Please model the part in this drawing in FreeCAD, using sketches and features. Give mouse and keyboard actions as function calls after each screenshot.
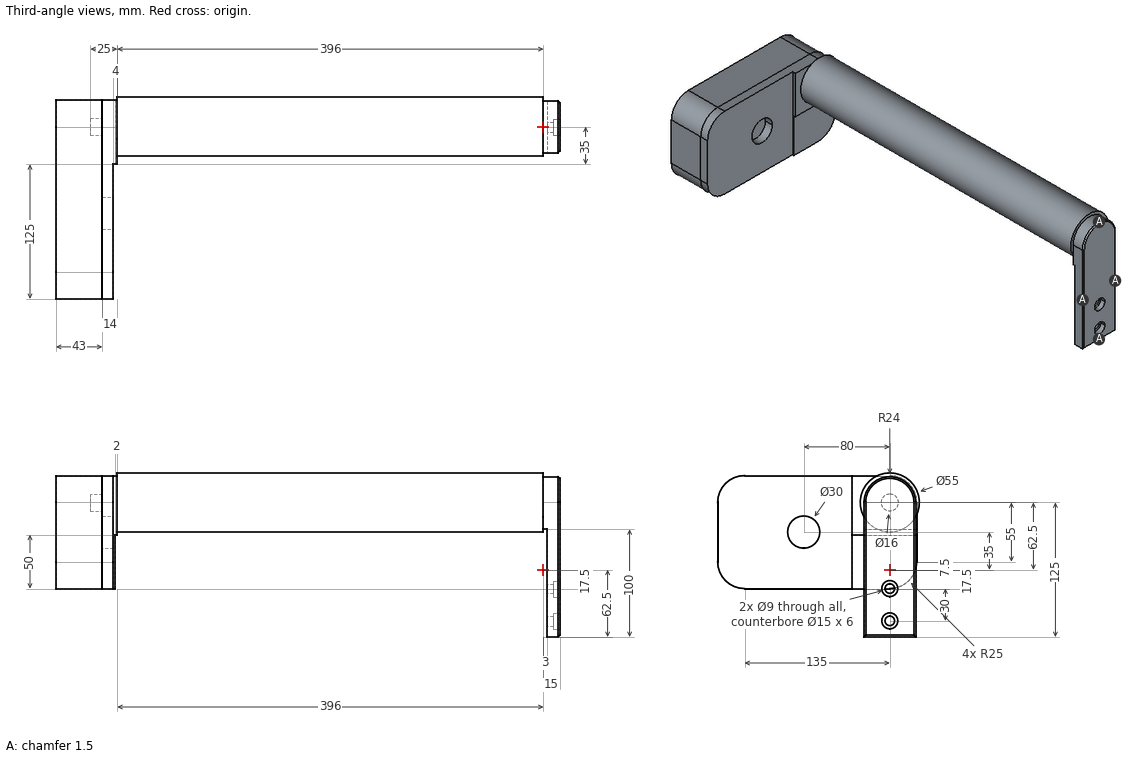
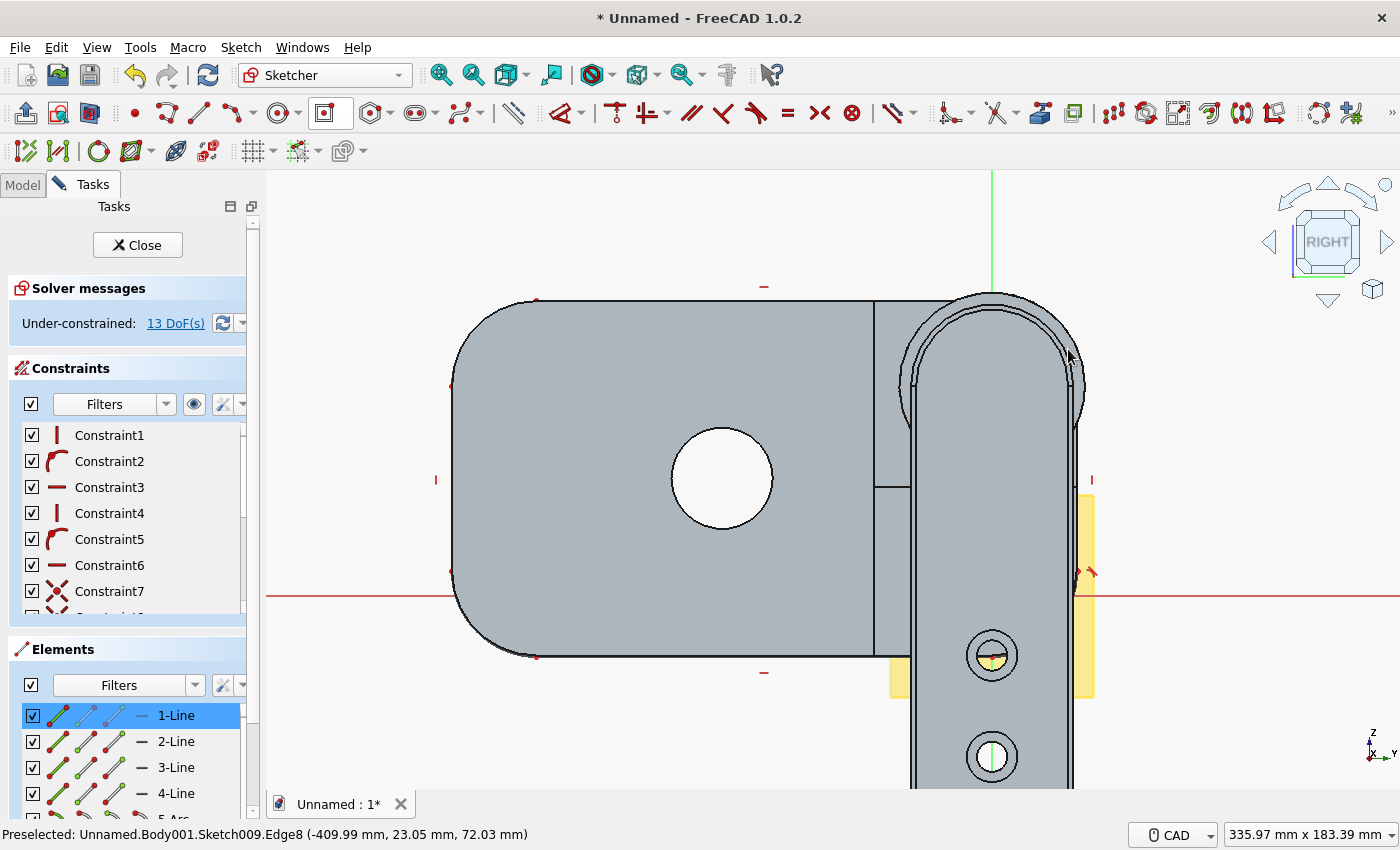
key(t)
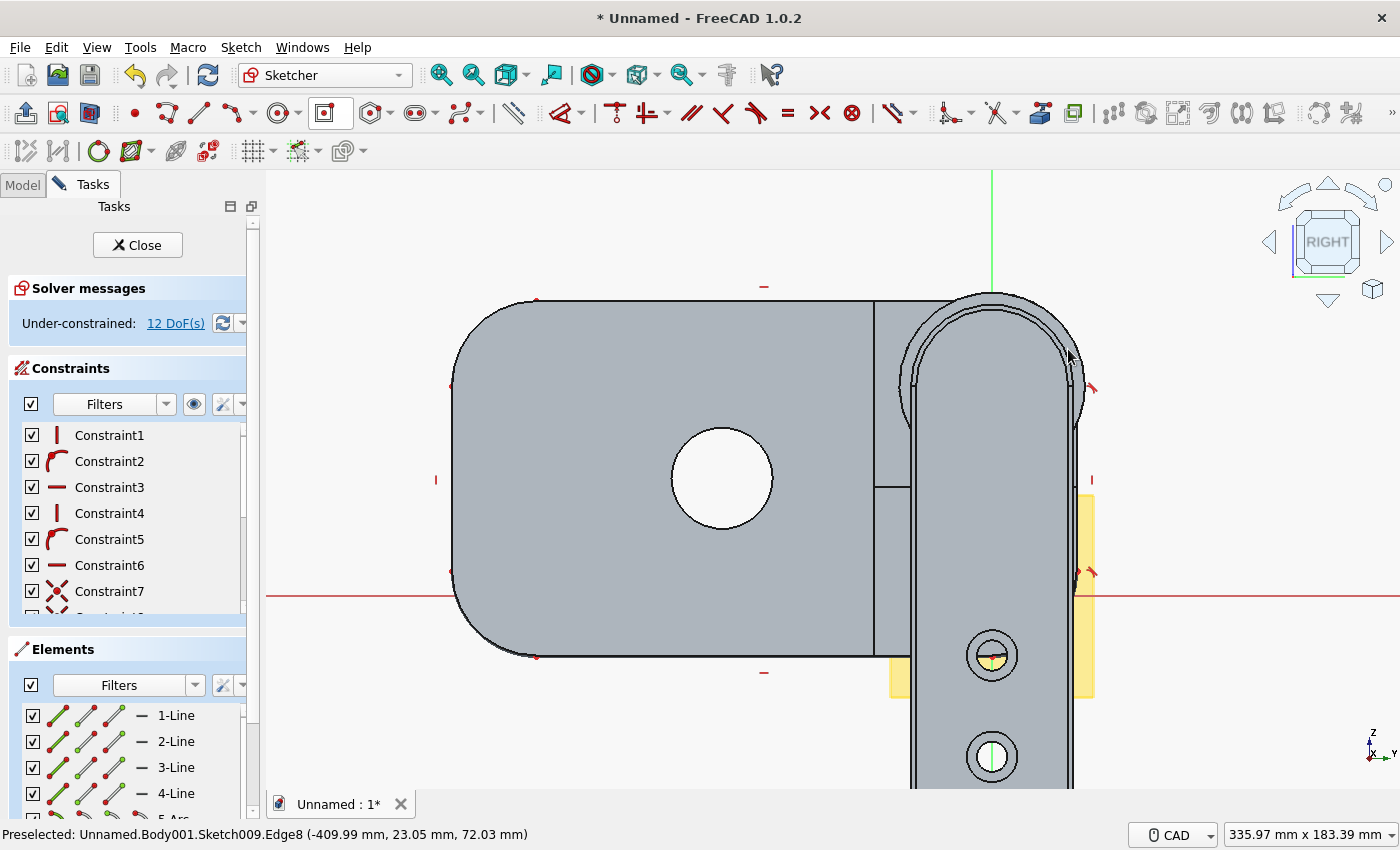
click(855, 657)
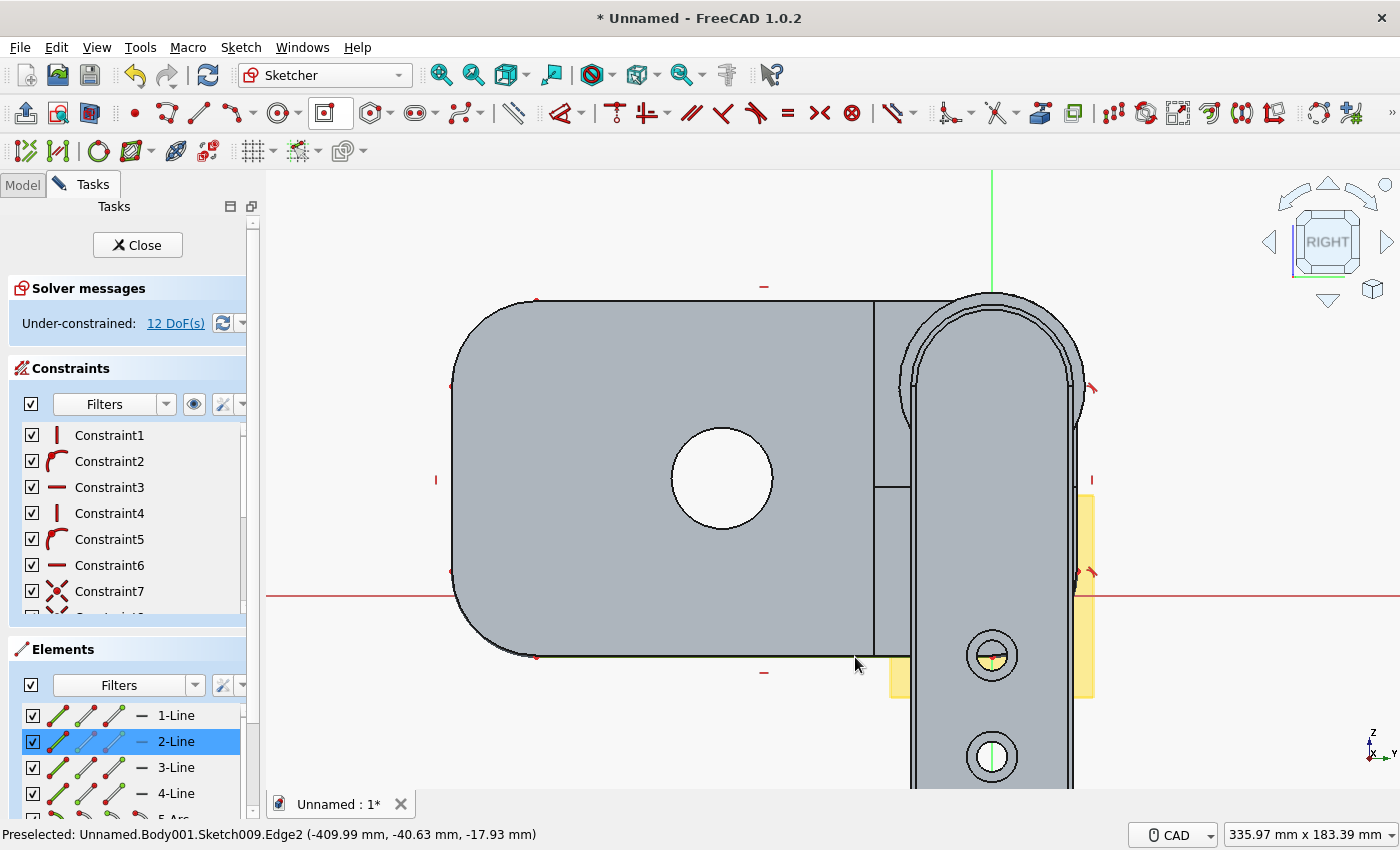
click(1031, 648)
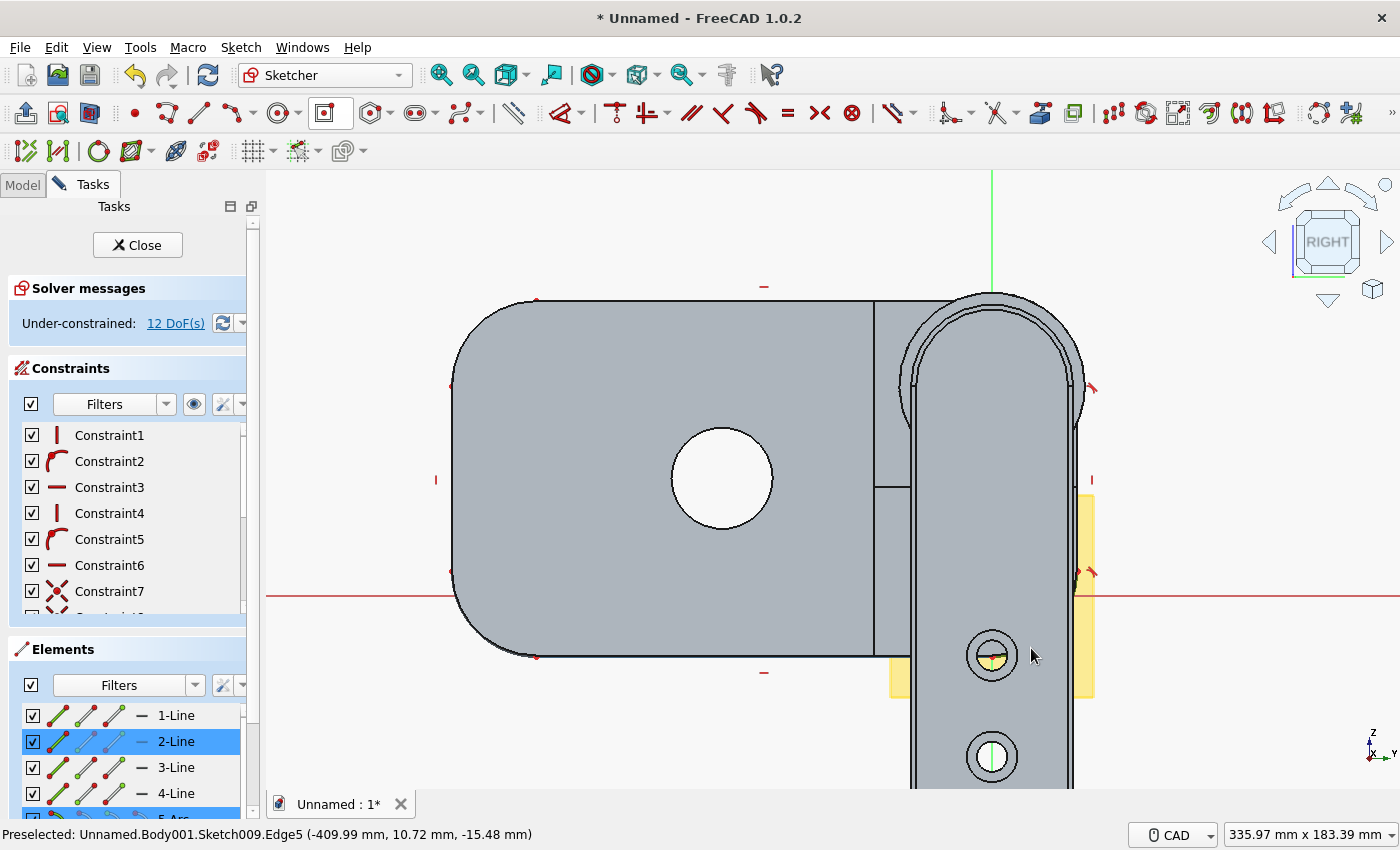
key(t)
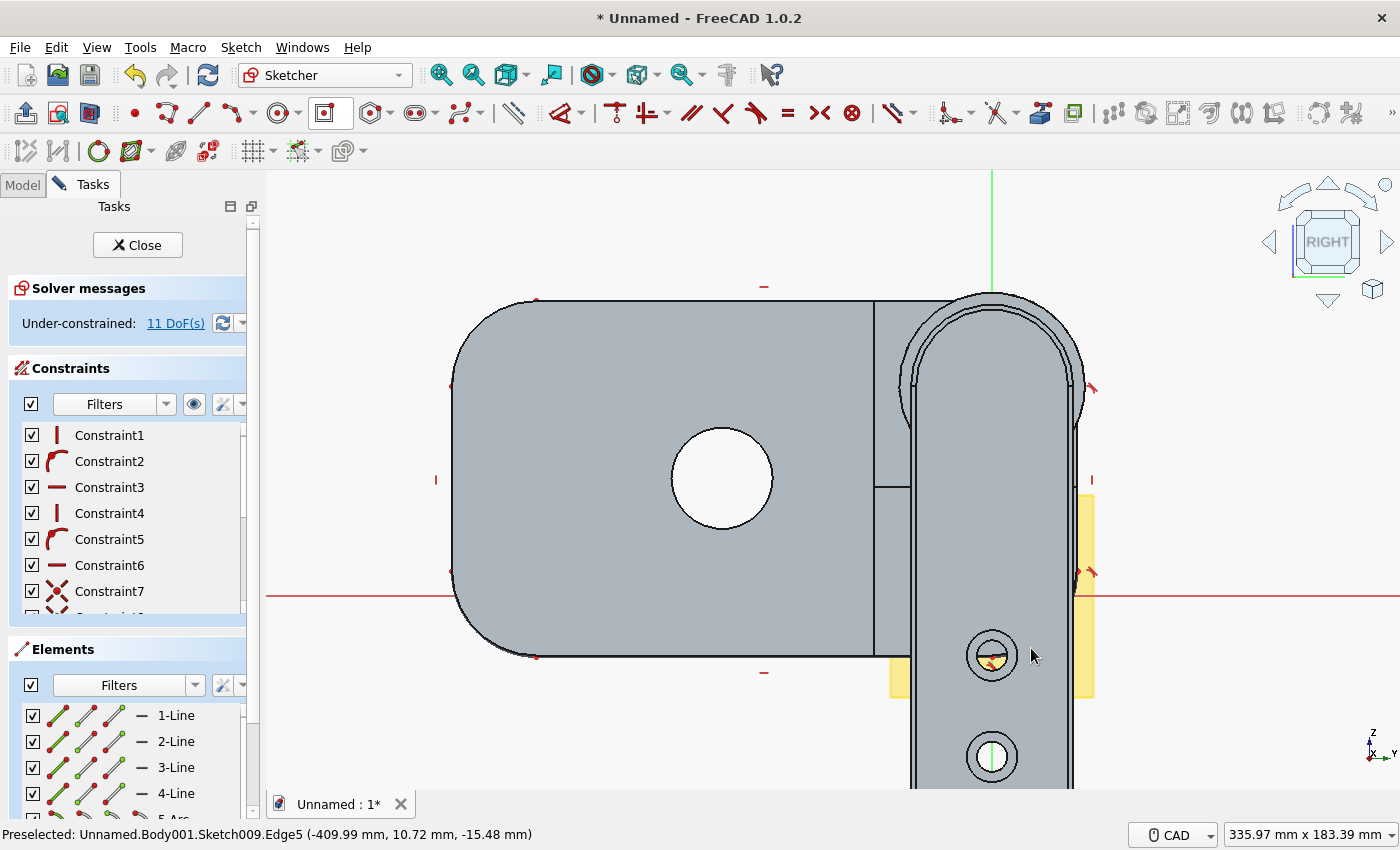
click(855, 657)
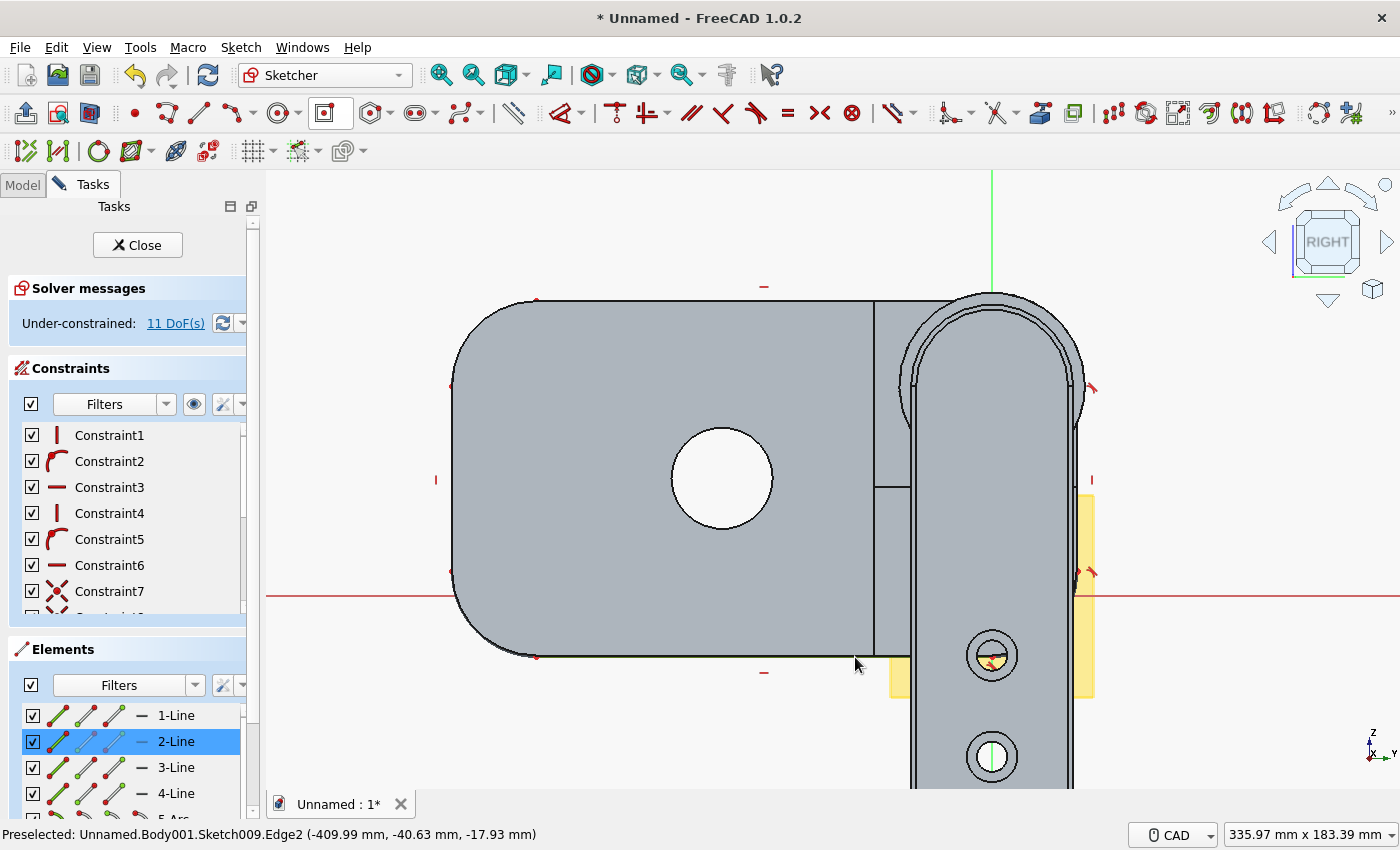
click(461, 610)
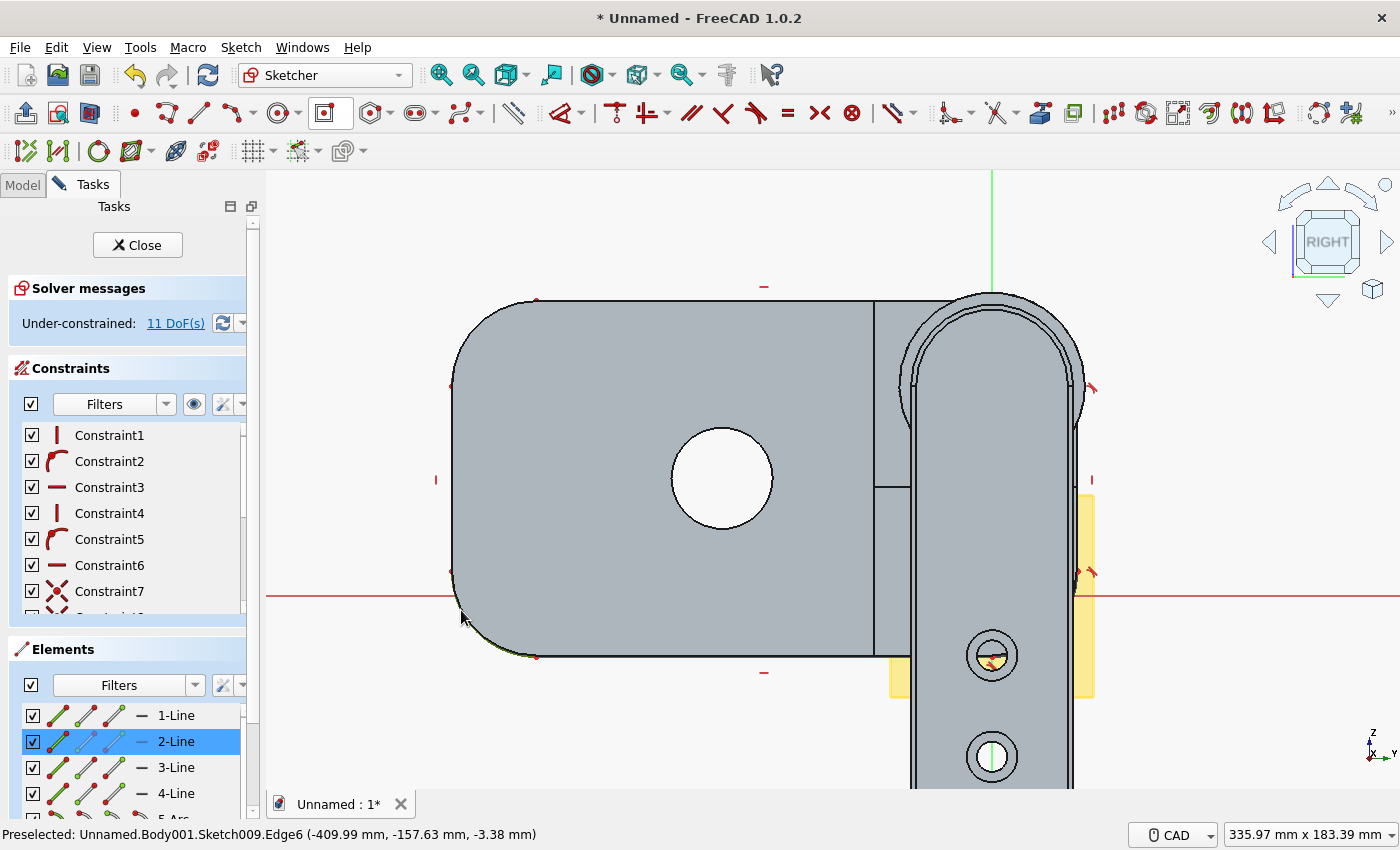
click(756, 114)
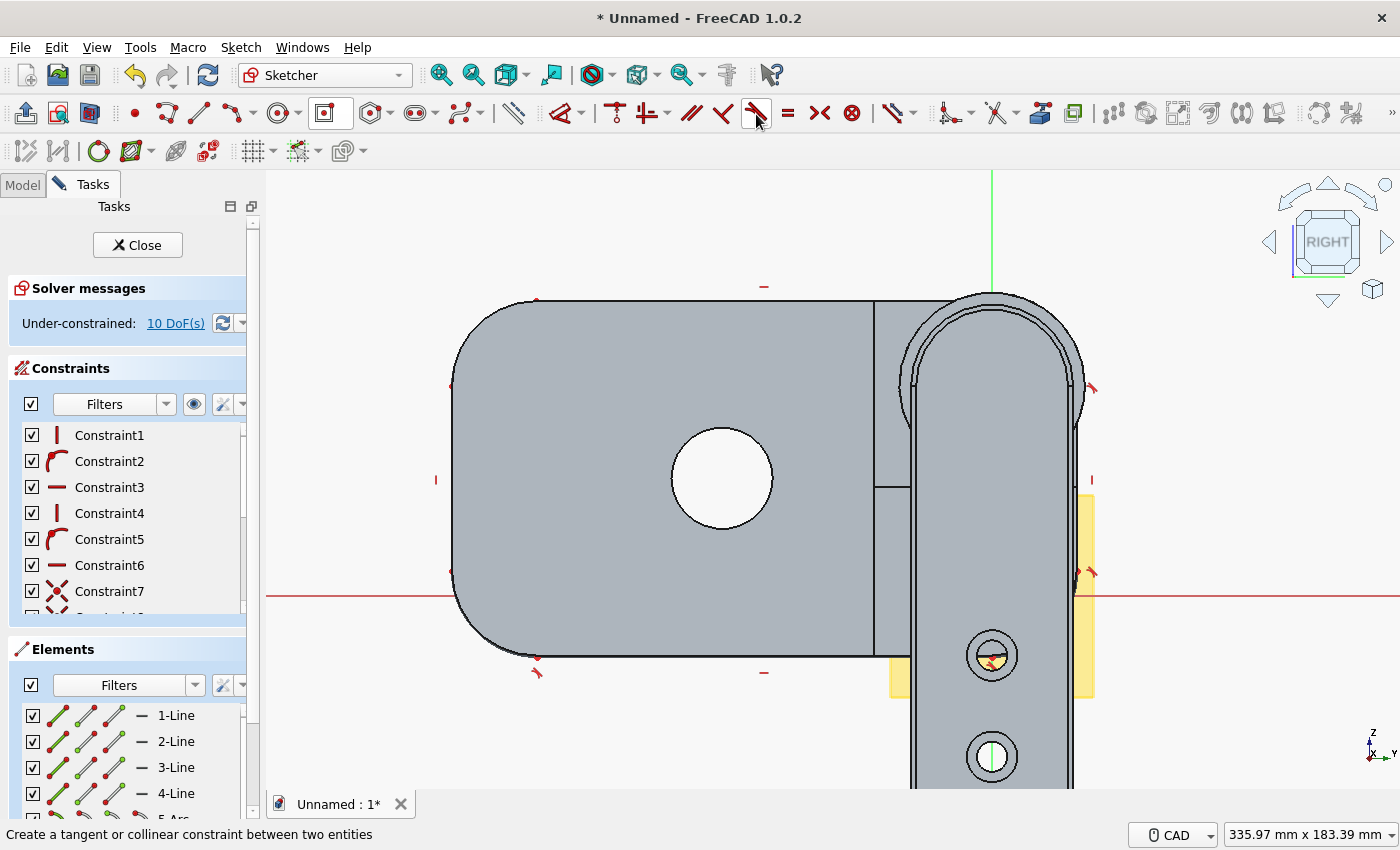
click(452, 516)